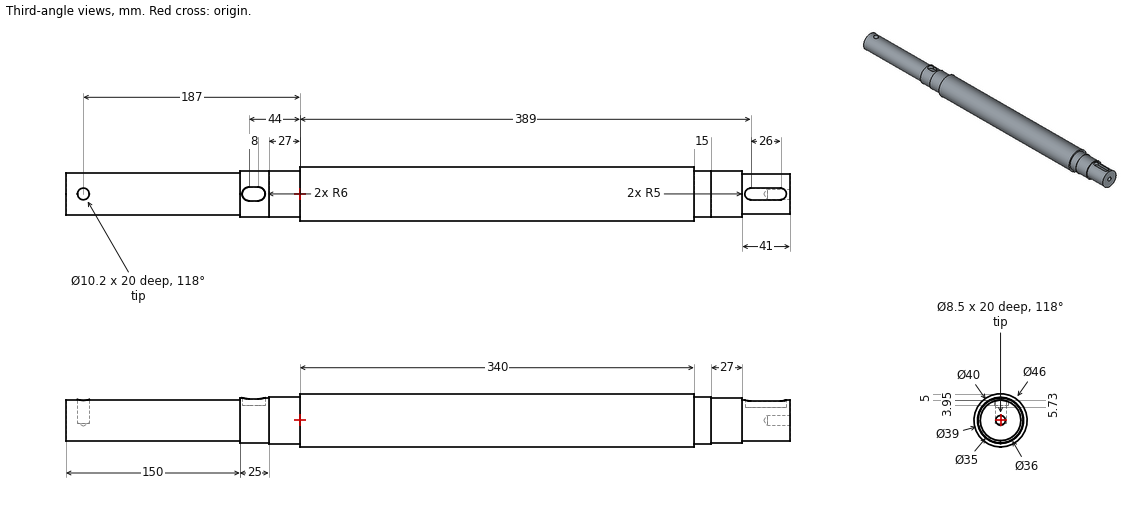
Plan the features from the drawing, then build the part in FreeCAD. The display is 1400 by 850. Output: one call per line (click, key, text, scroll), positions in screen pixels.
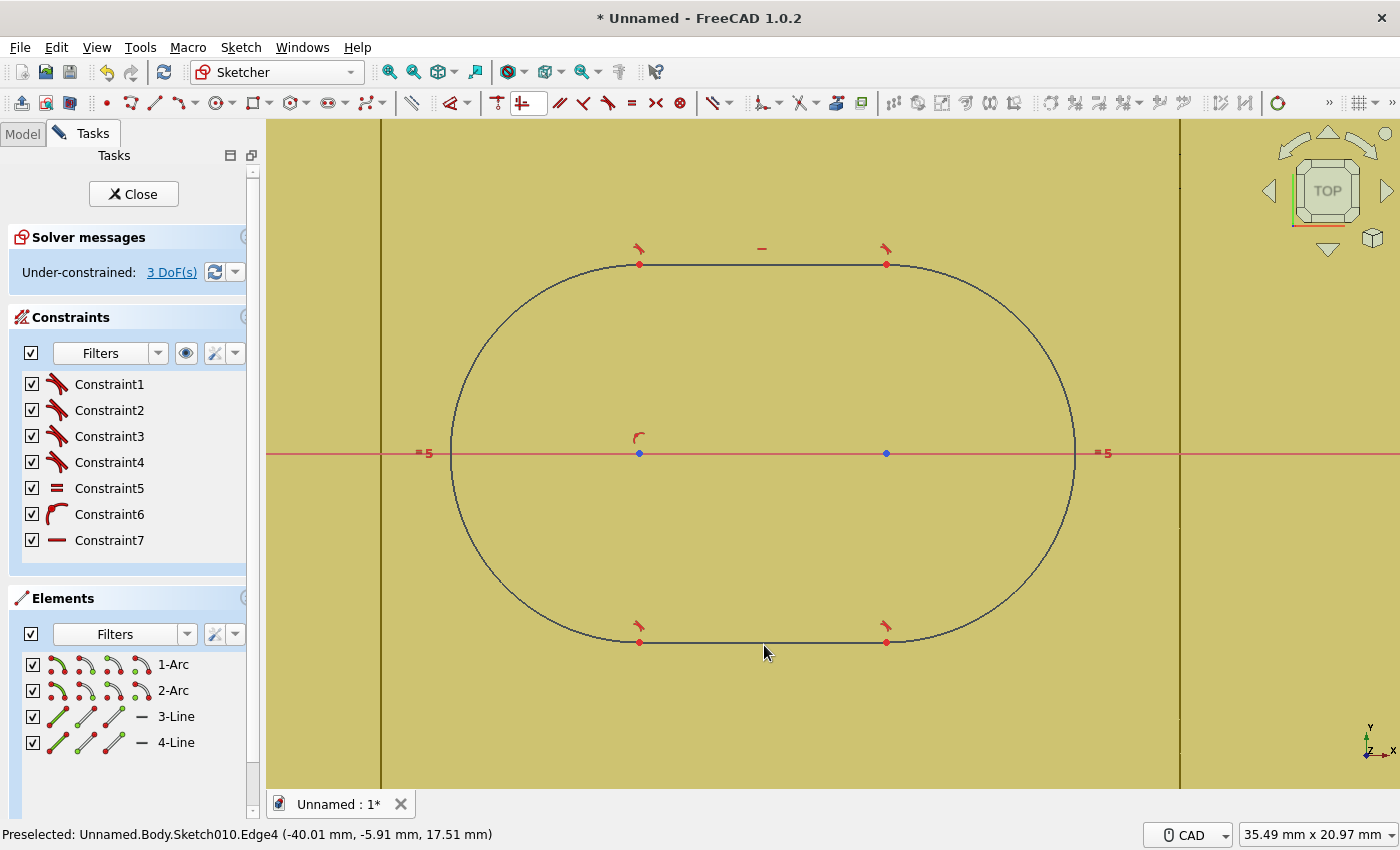
click(450, 104)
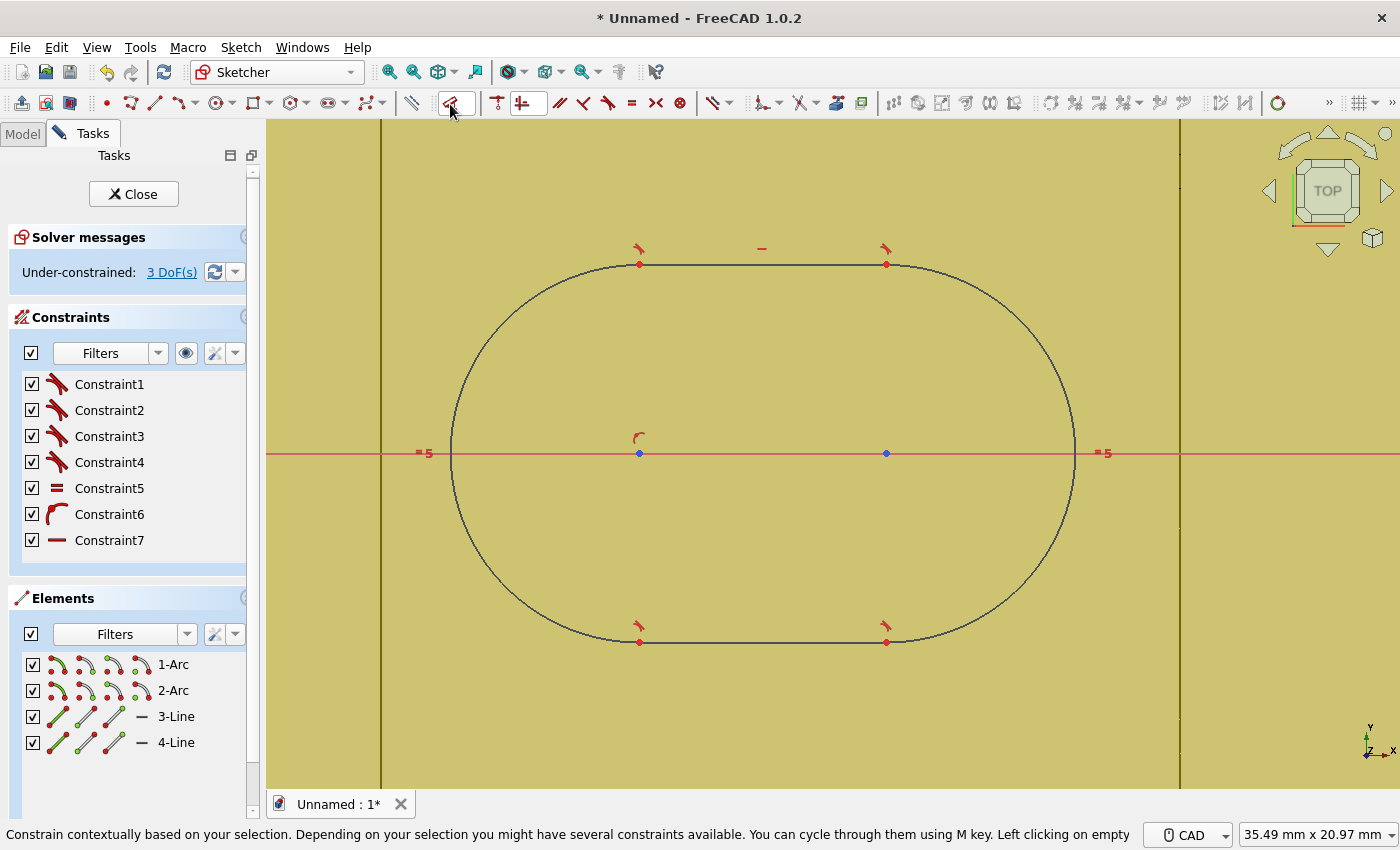
click(487, 343)
click(461, 324)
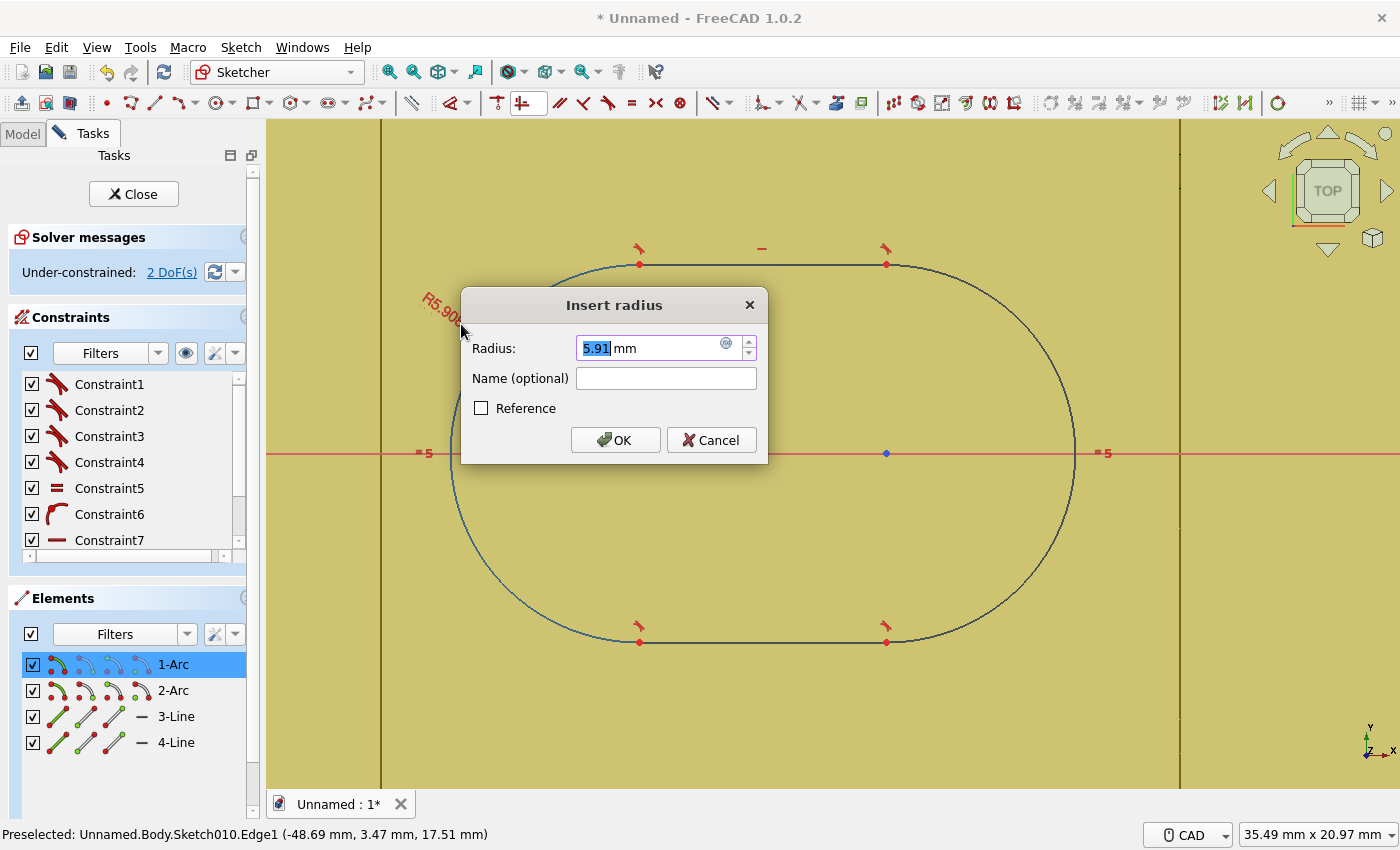
text(6)
key(Return)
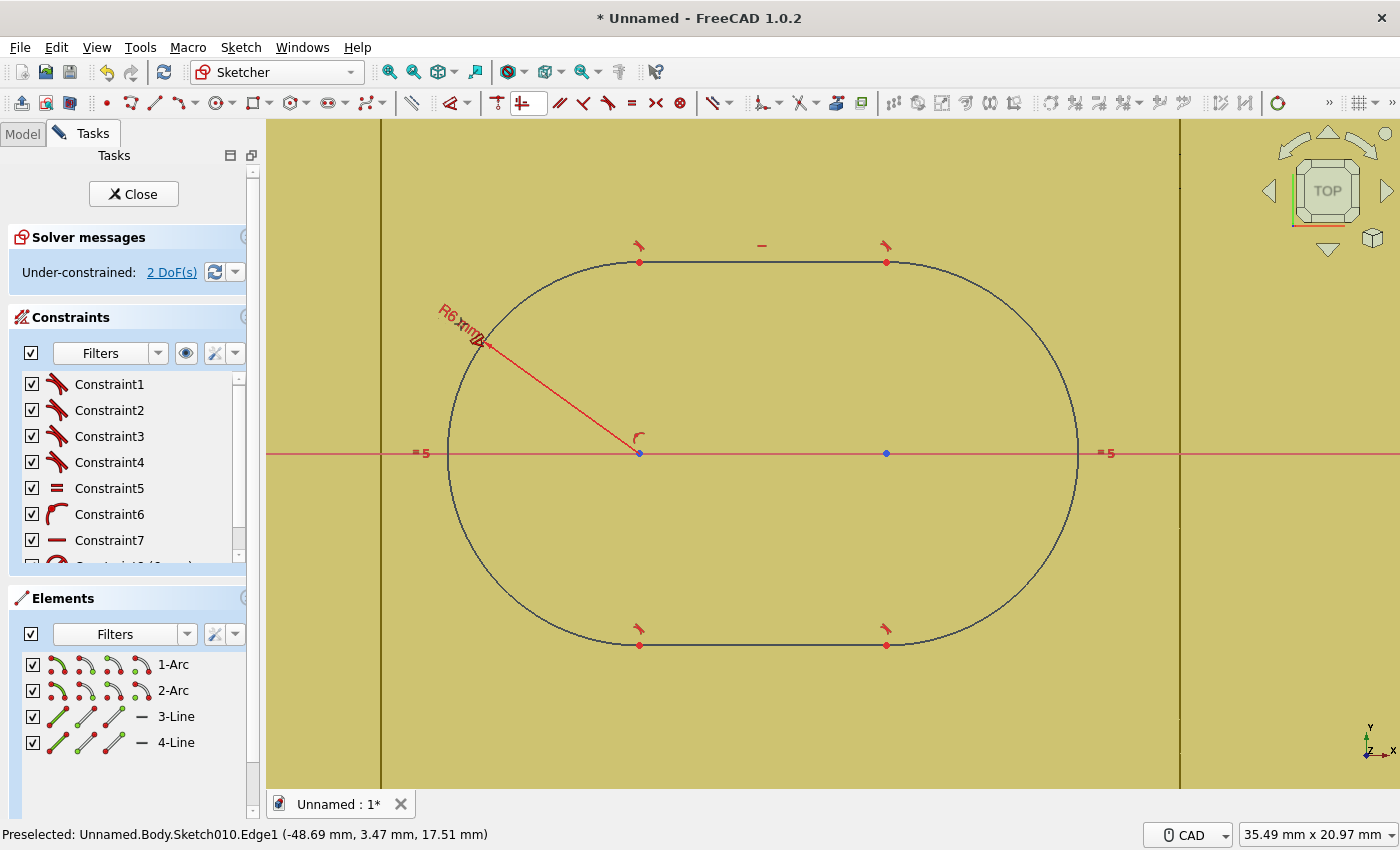
click(714, 262)
click(763, 228)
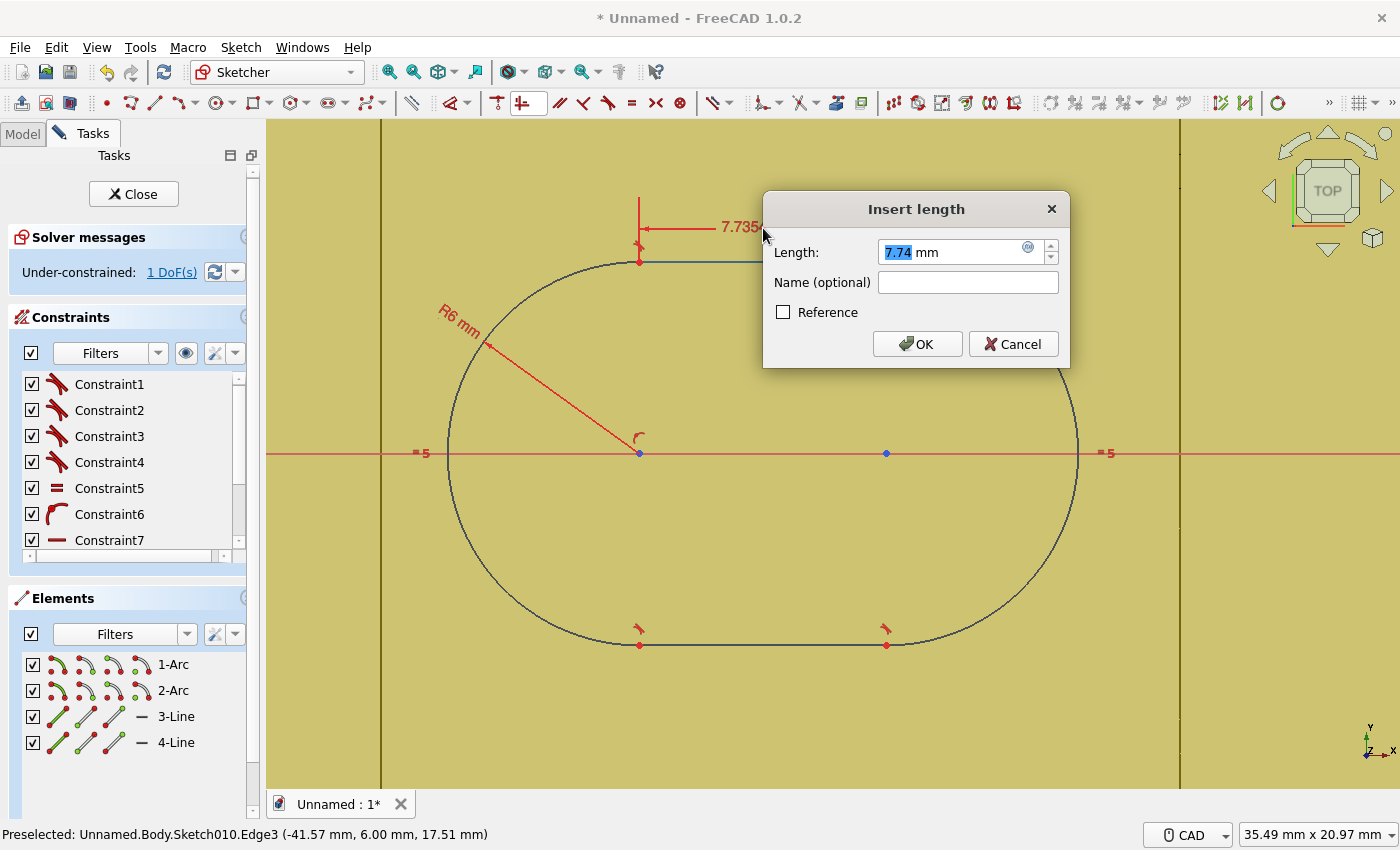
text(8)
key(Return)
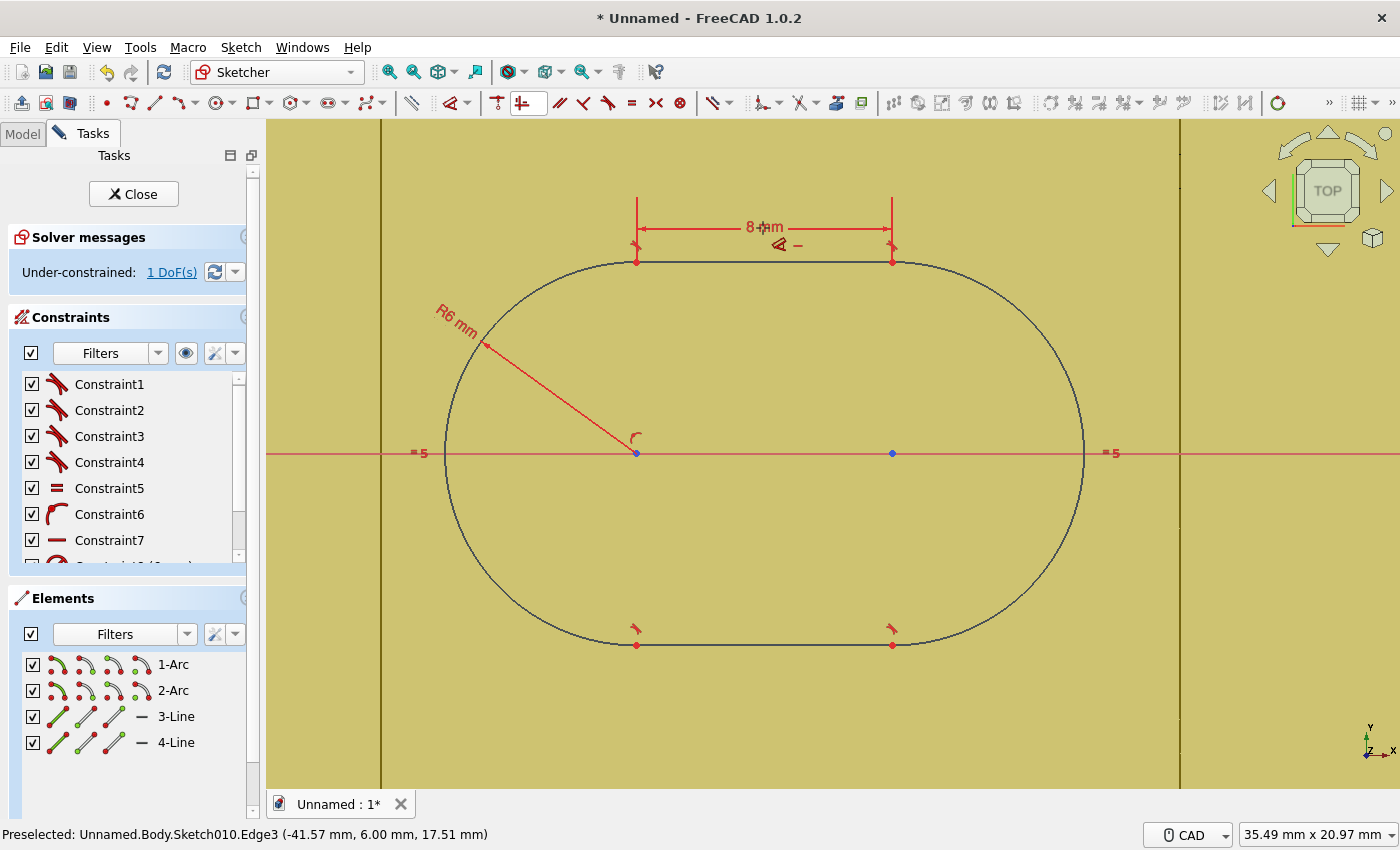
click(637, 262)
click(936, 228)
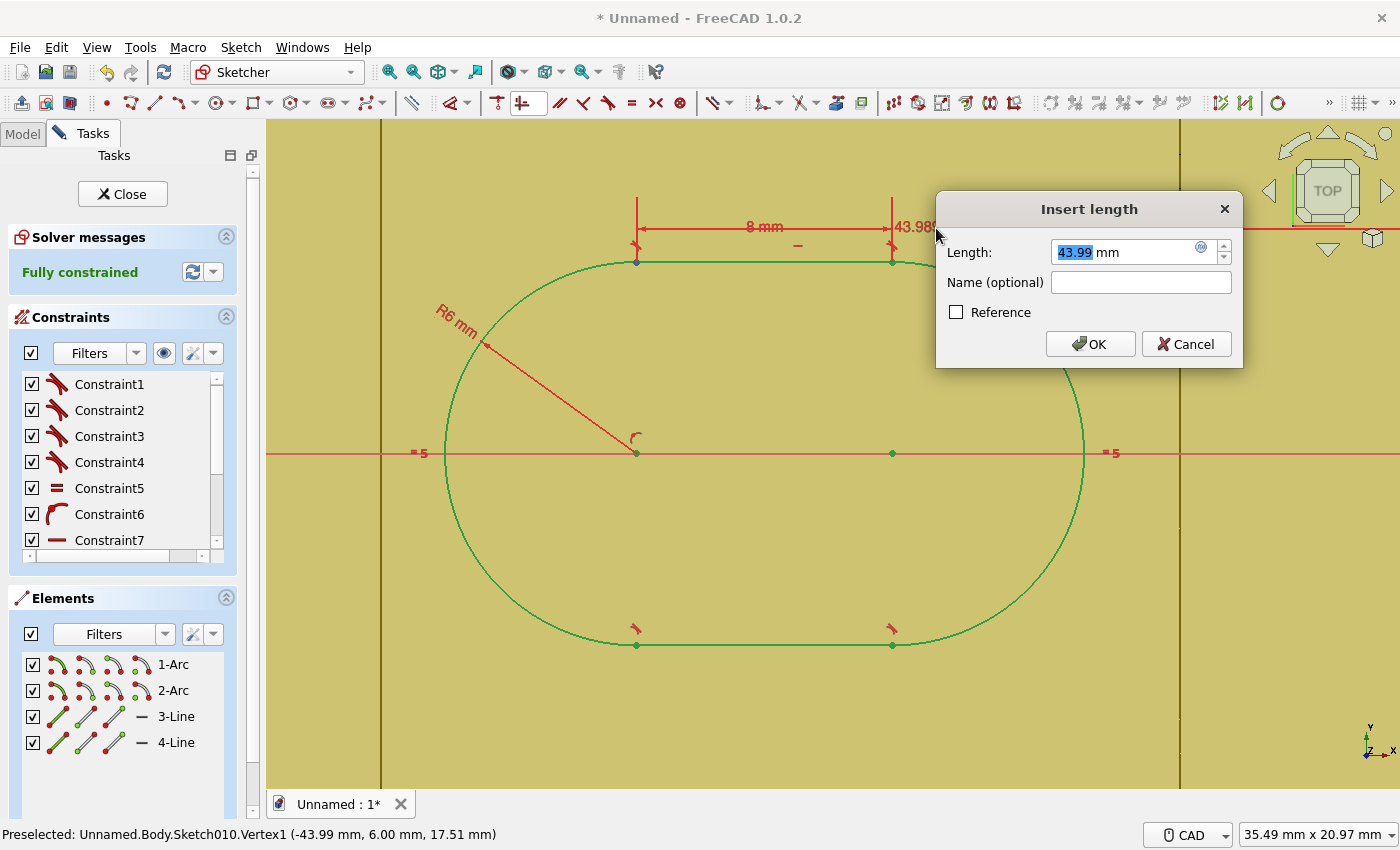
text(44)
key(Return)
key(Escape)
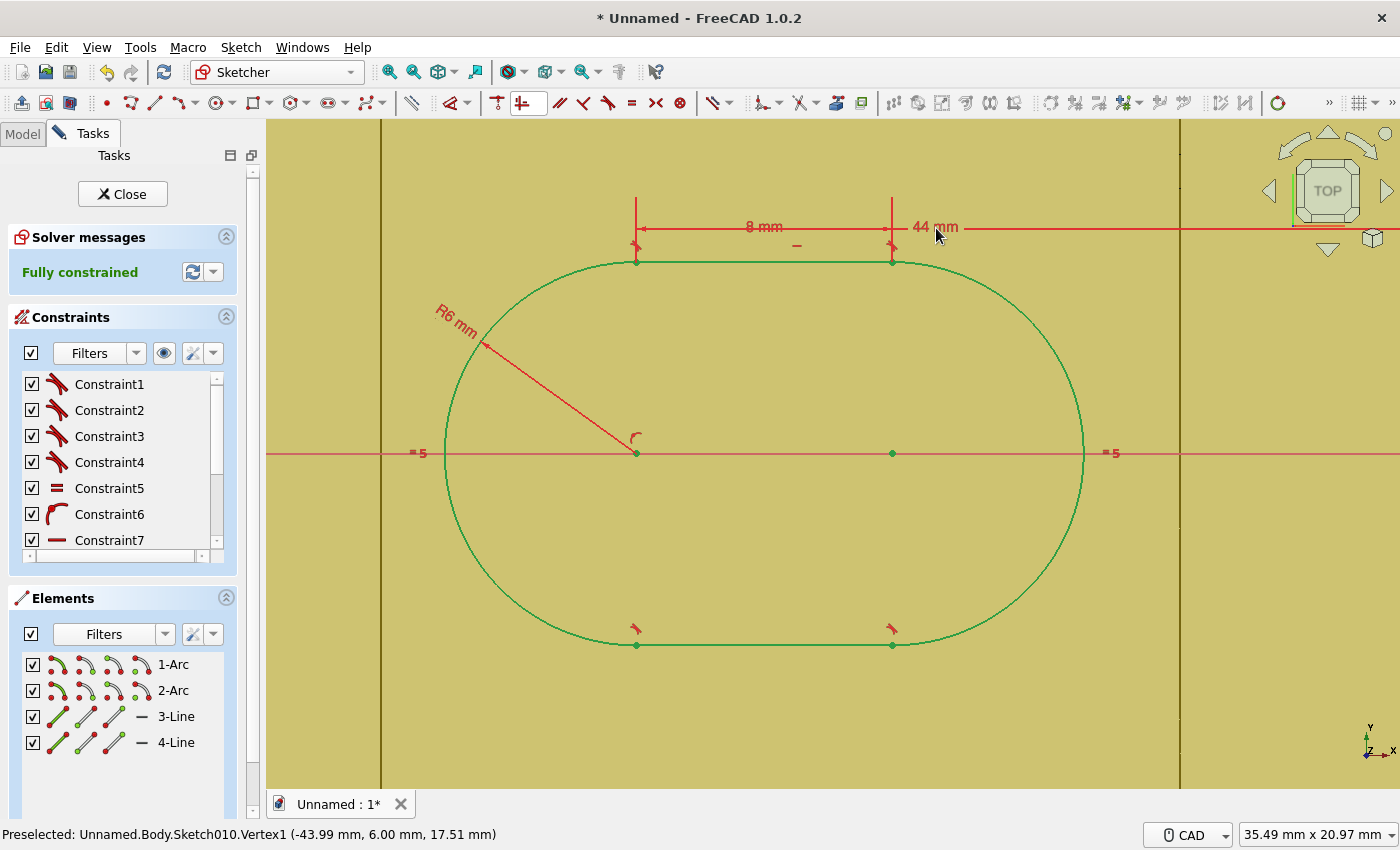
click(123, 194)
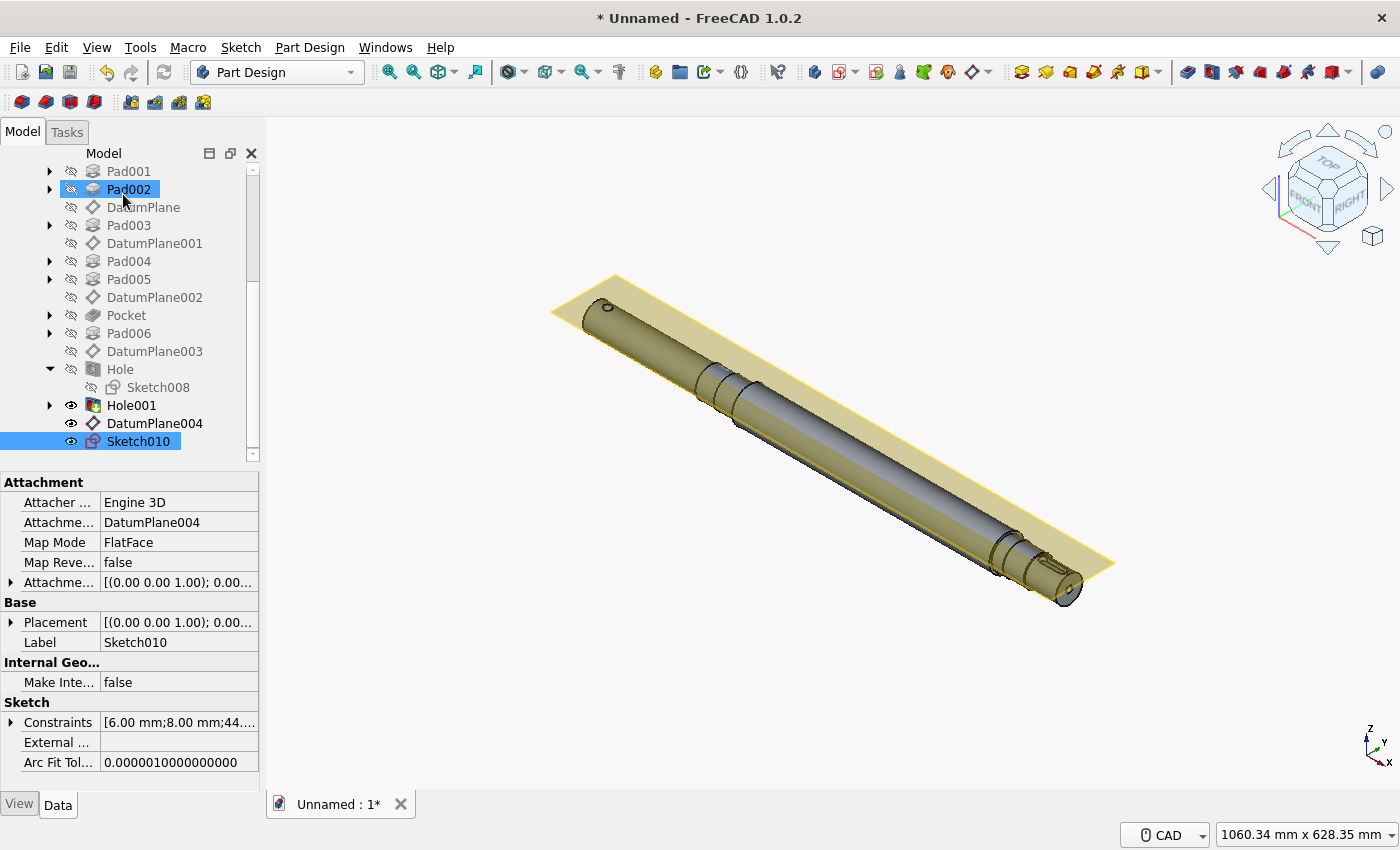
click(1188, 72)